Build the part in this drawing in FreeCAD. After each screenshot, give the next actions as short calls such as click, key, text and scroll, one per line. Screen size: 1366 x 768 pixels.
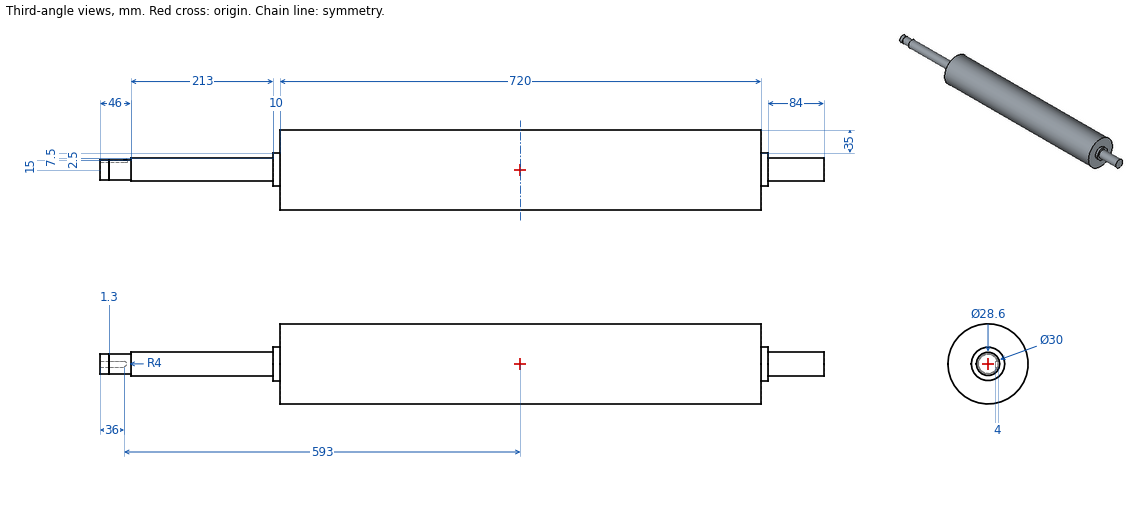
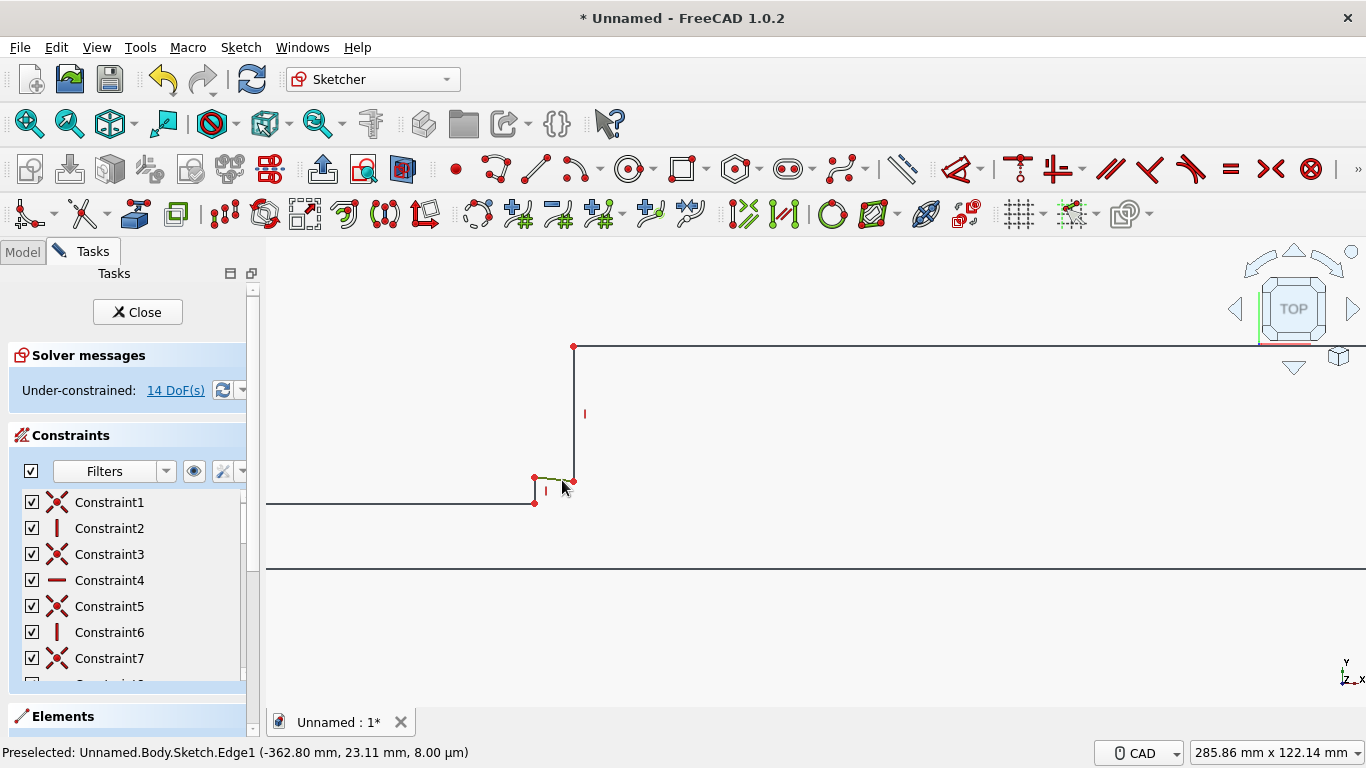
key(h)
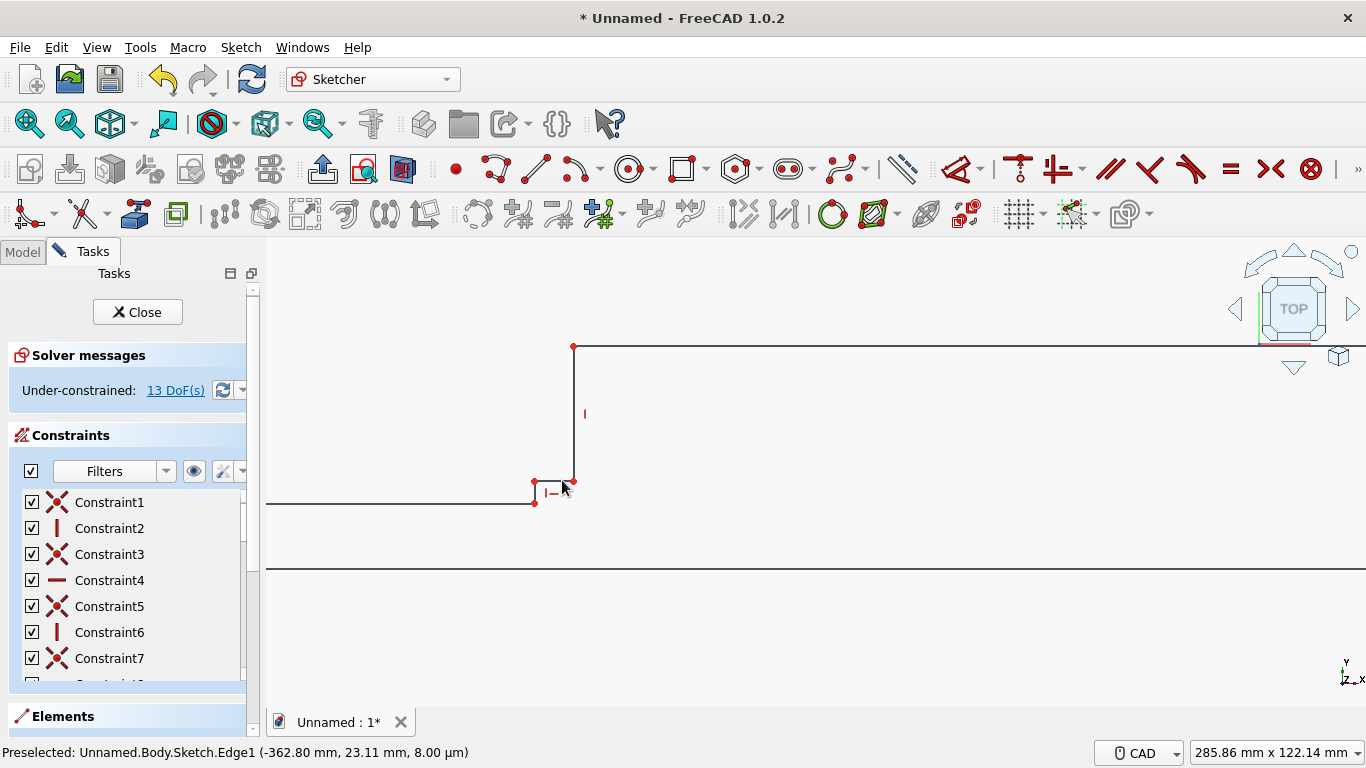
click(535, 504)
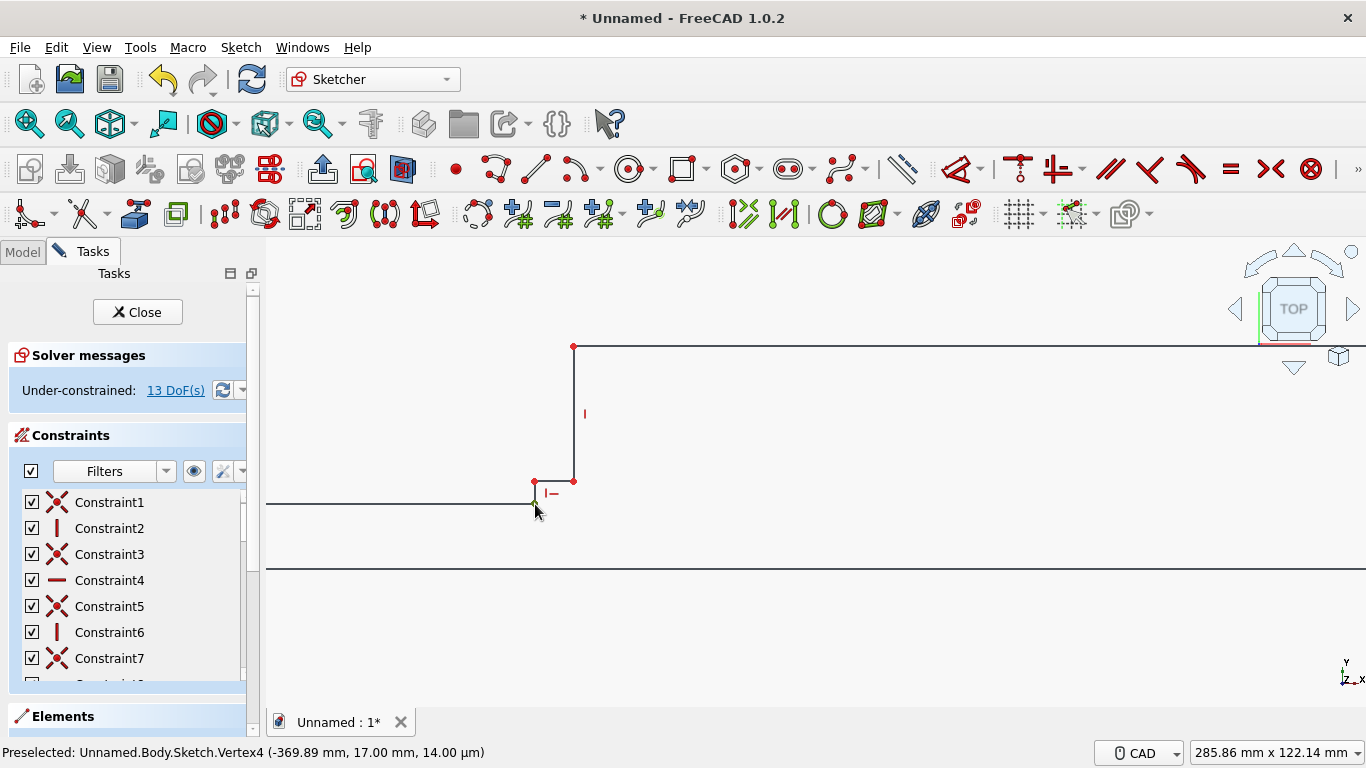
scroll(574, 476, down, 9)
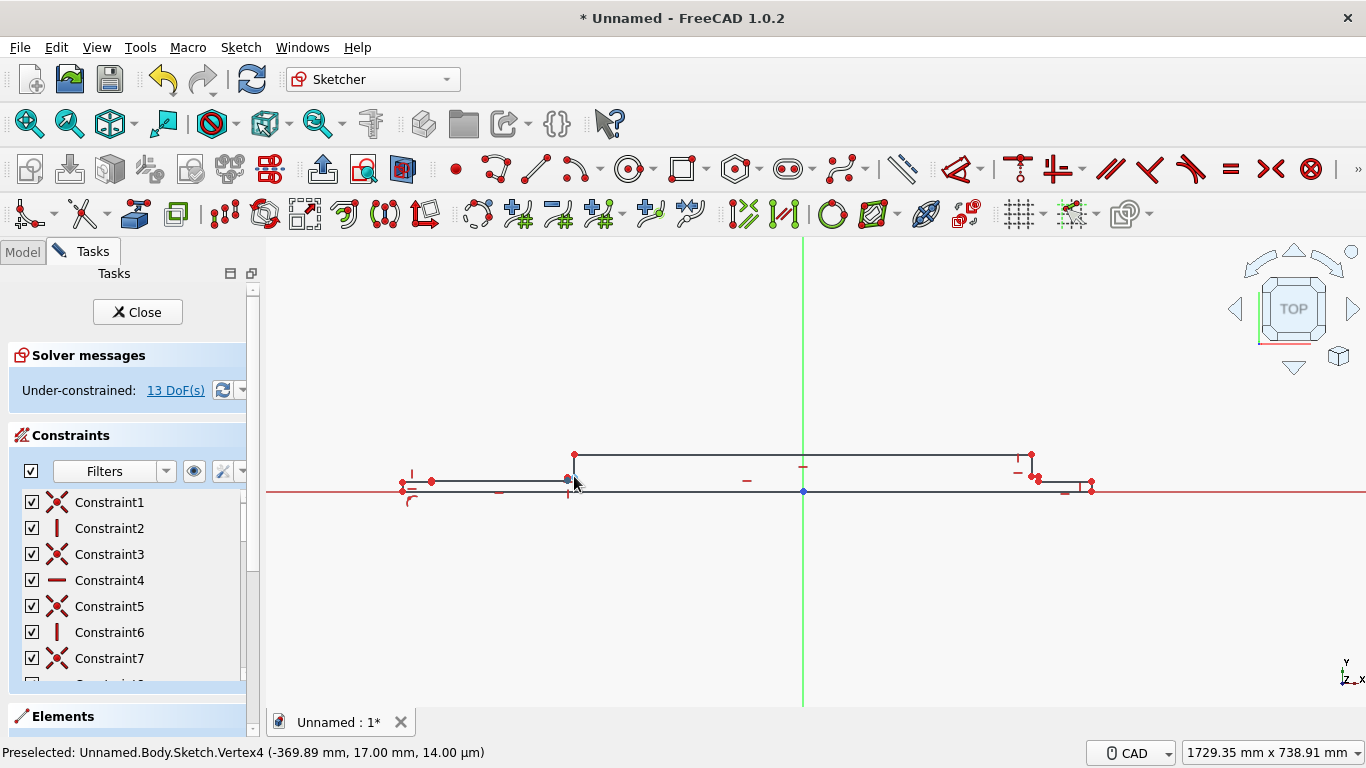
scroll(1039, 482, up, 5)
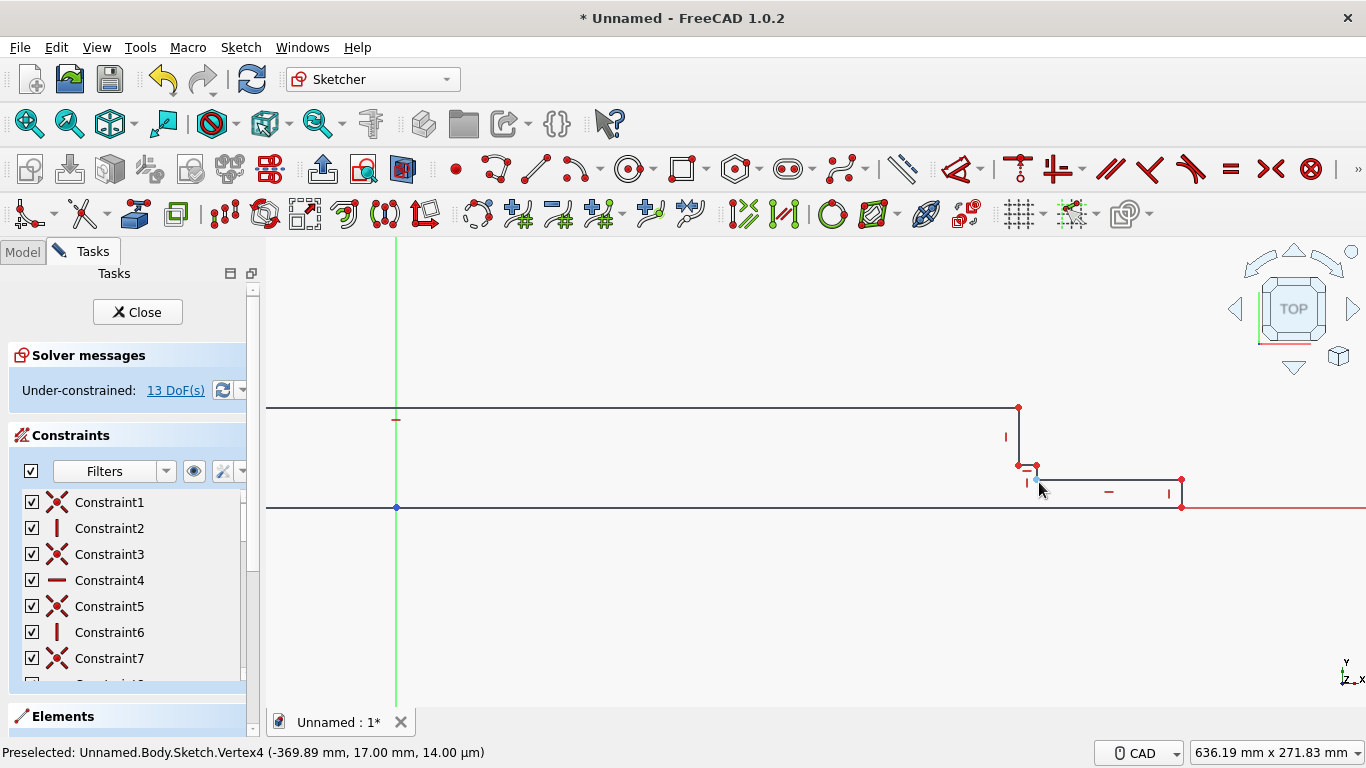
click(1037, 480)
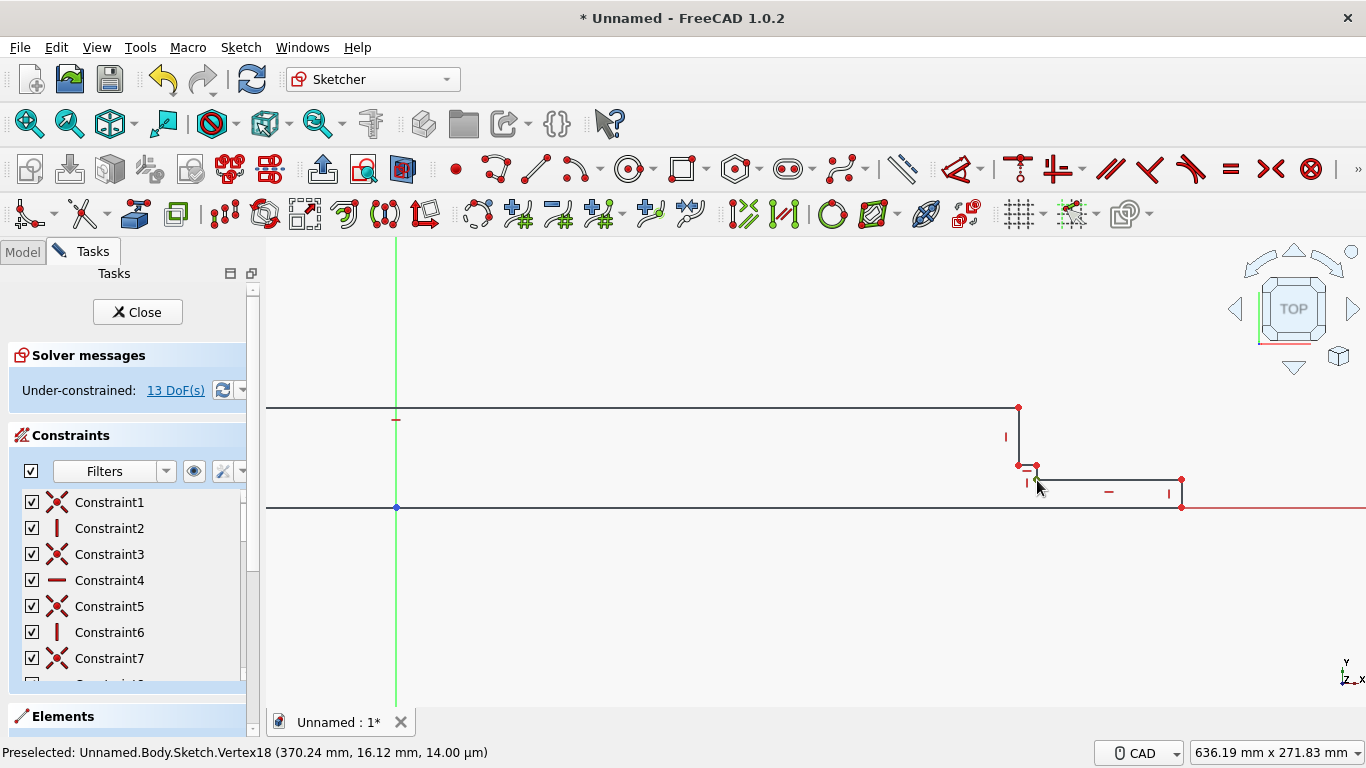
click(396, 649)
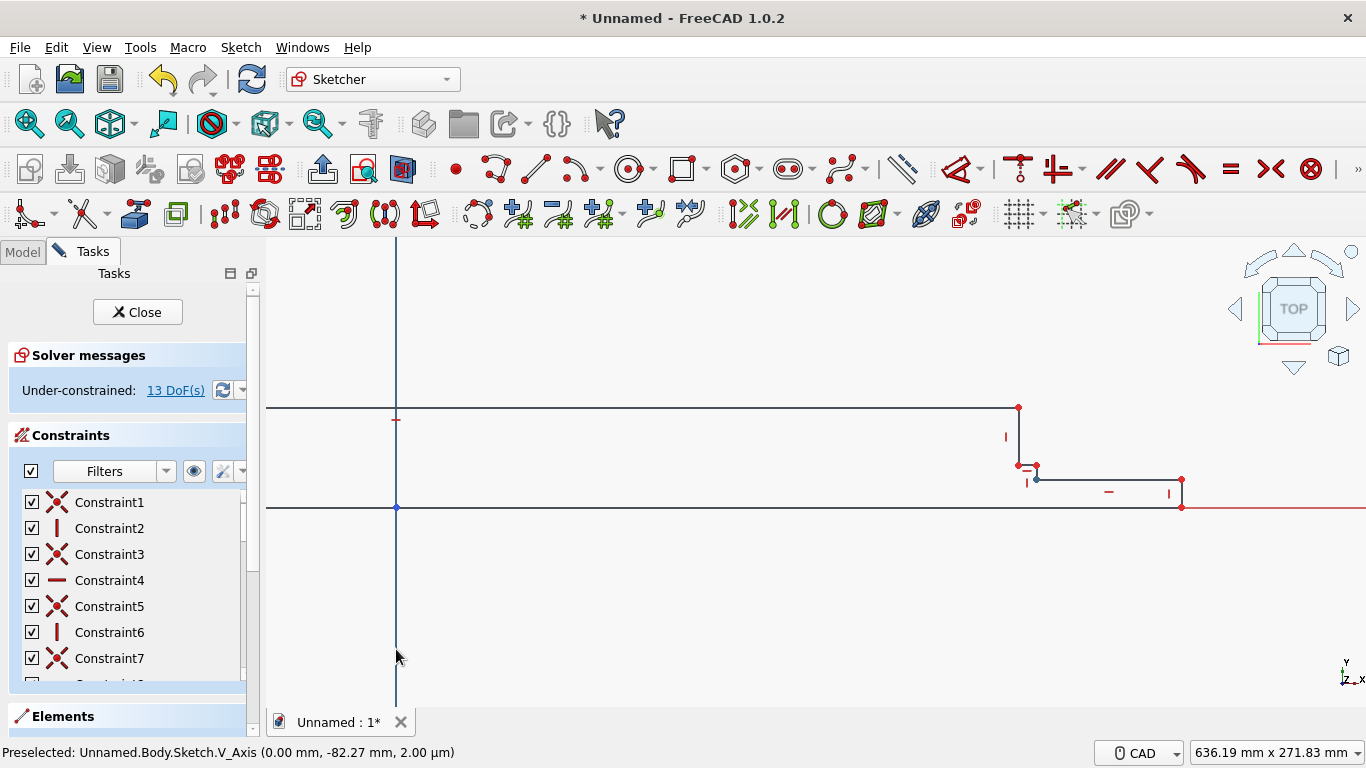
click(1272, 170)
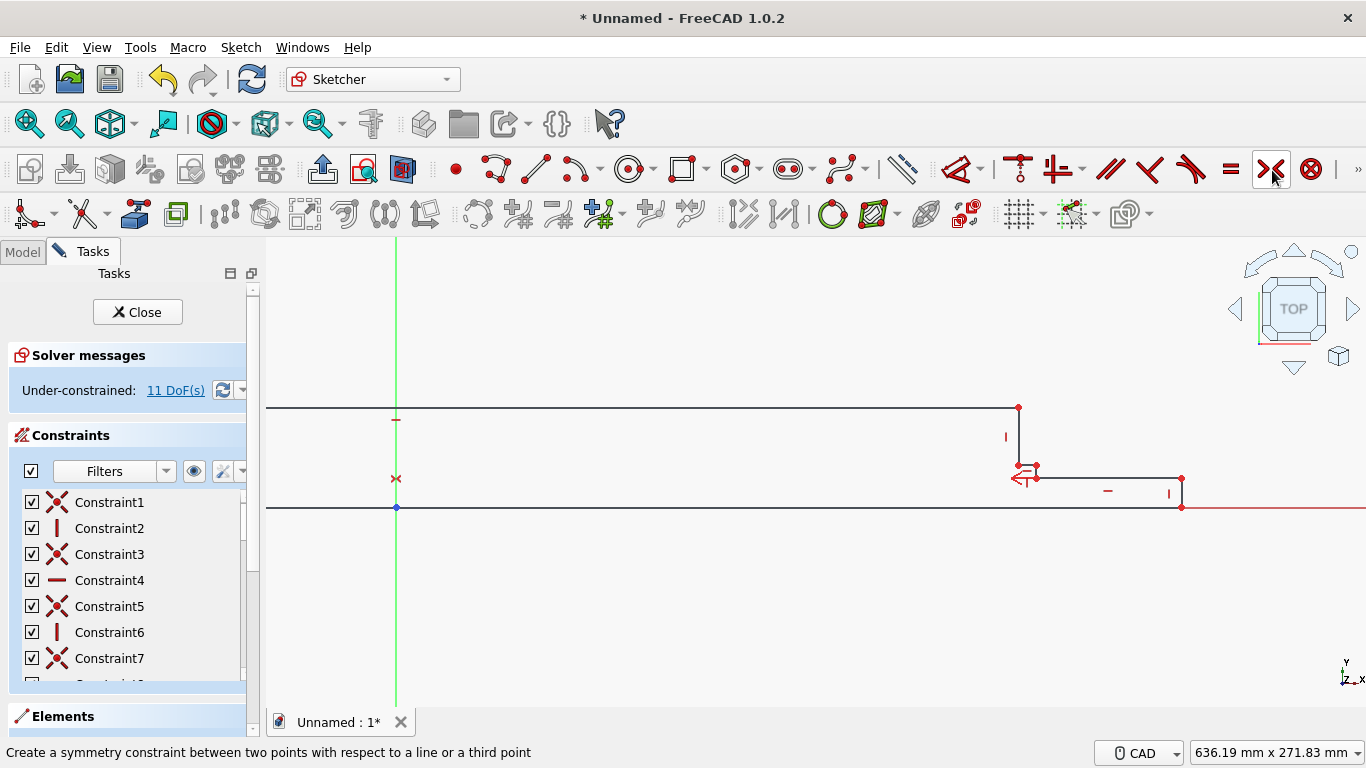
scroll(1040, 481, down, 5)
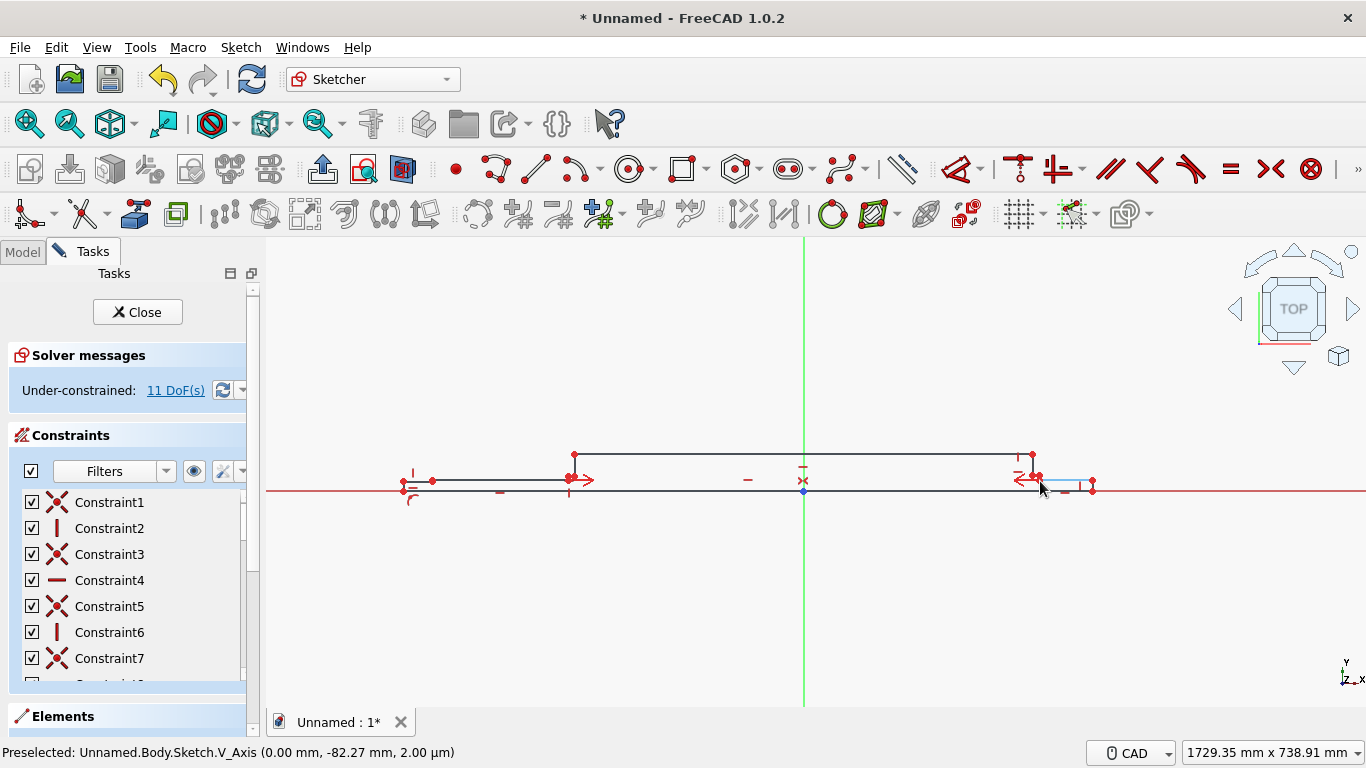
scroll(575, 477, up, 4)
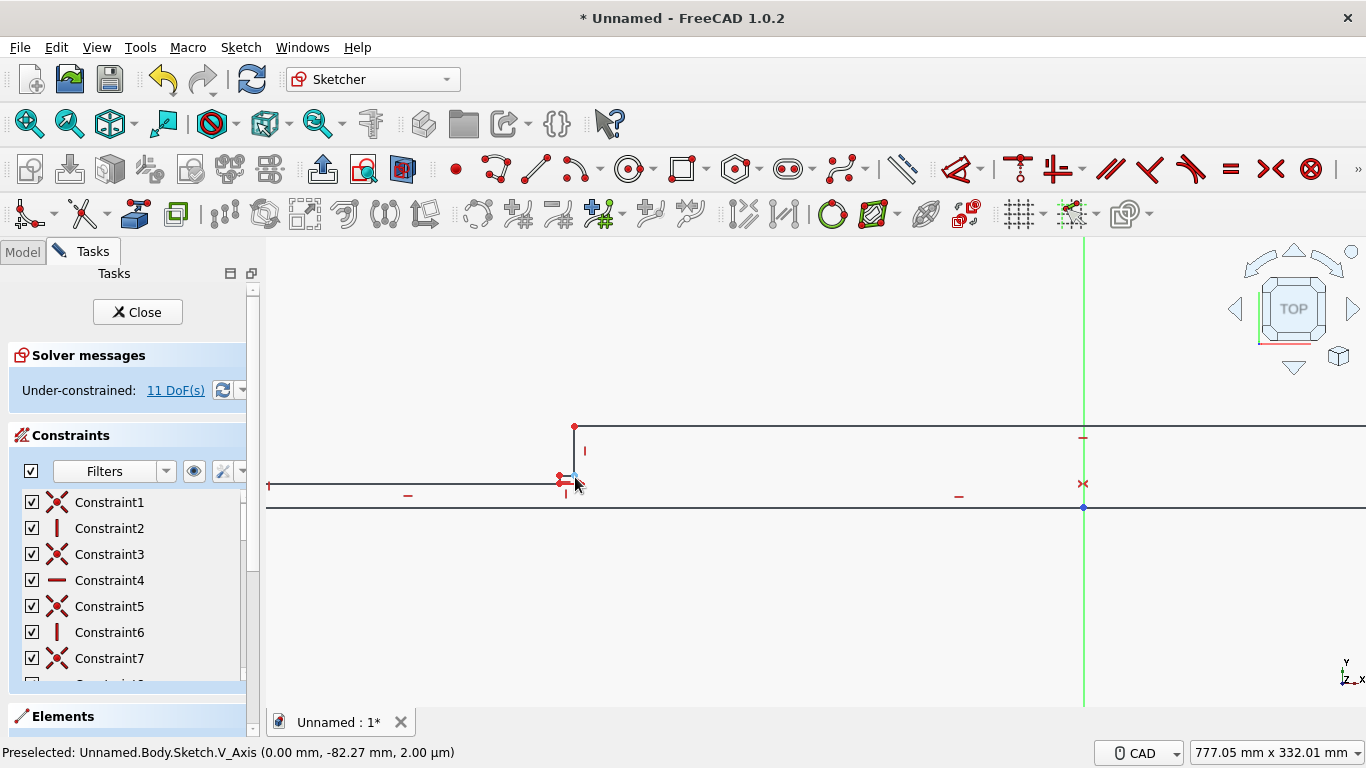
click(574, 476)